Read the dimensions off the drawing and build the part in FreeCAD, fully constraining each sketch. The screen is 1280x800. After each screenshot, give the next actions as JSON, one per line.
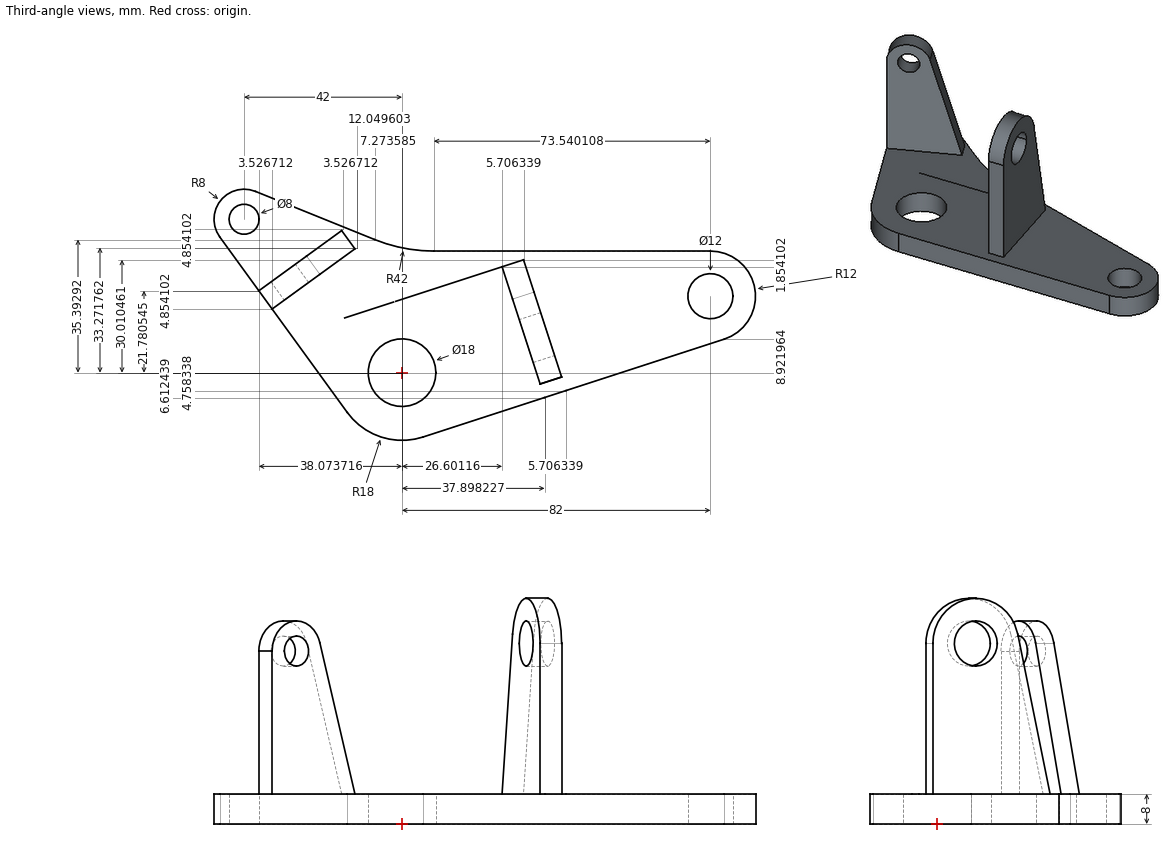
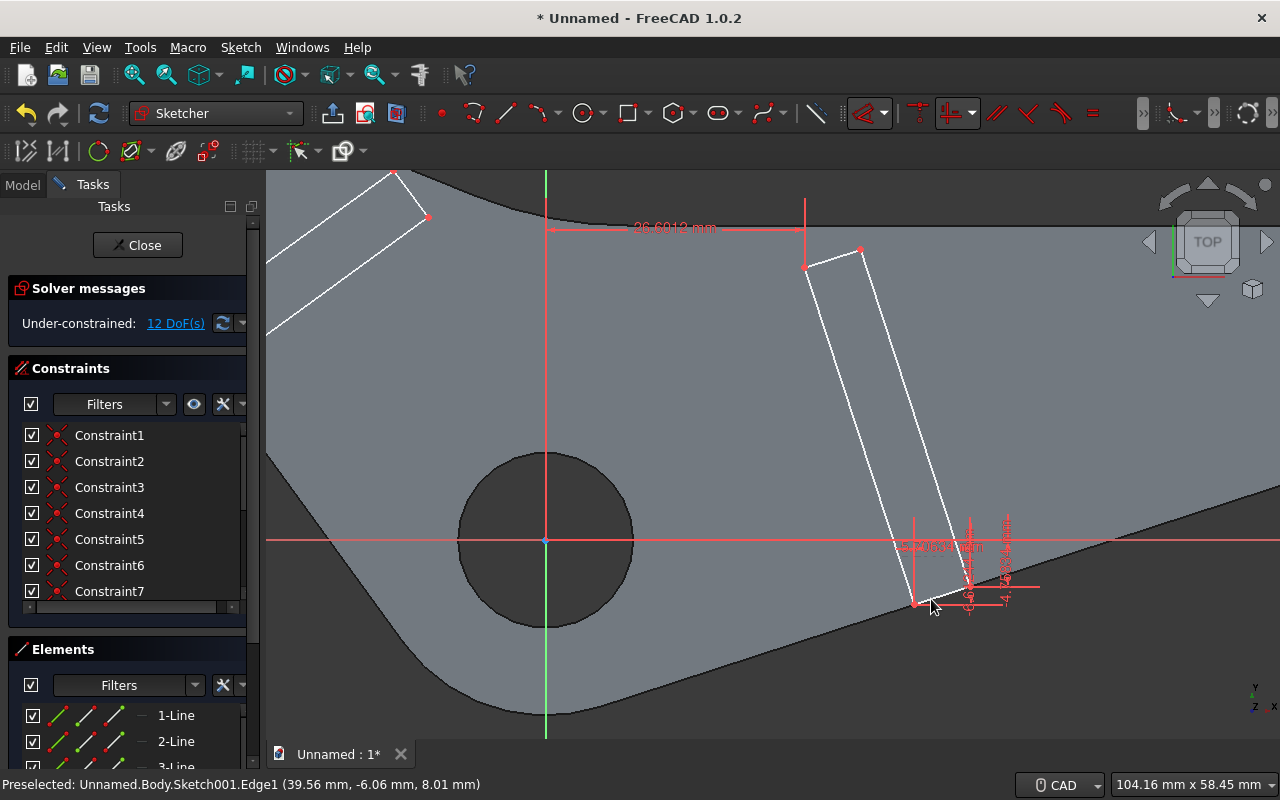
{"action": "left_click", "coordinate": [844, 255]}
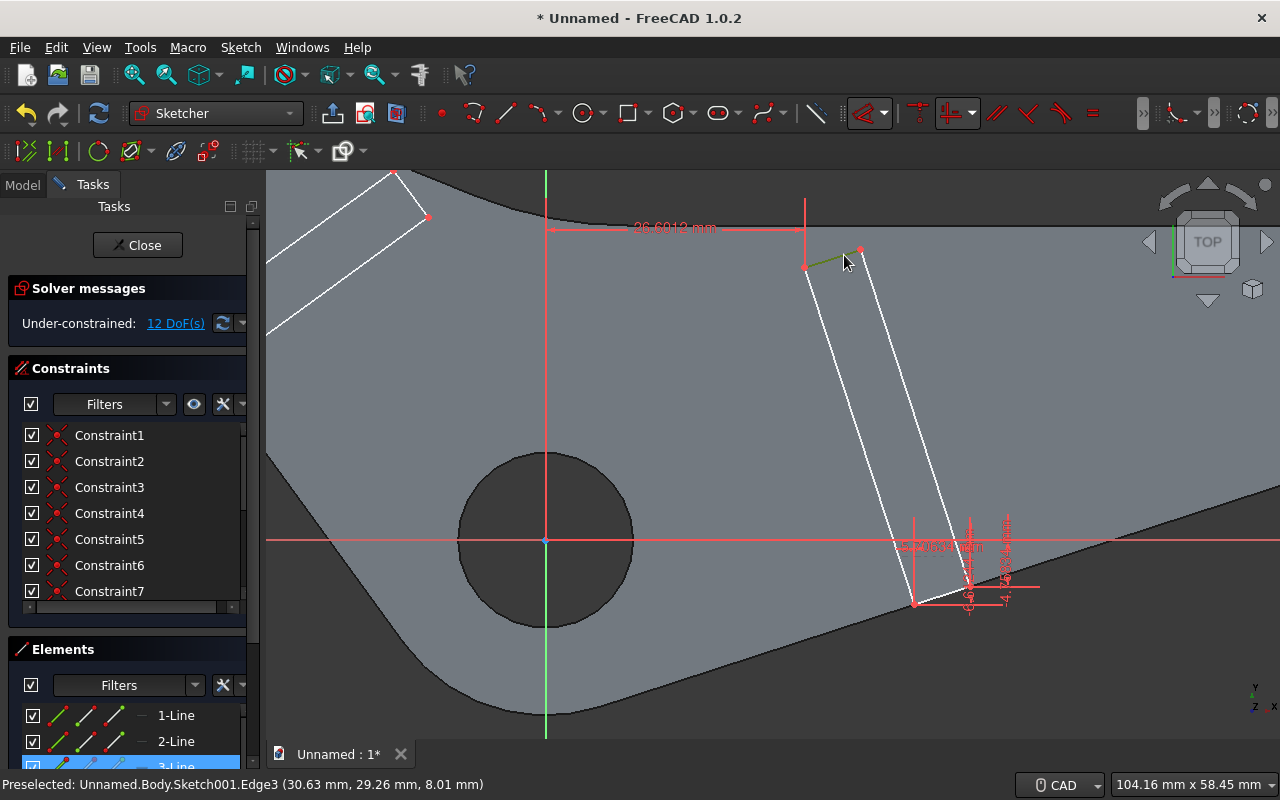
{"action": "key", "text": "l"}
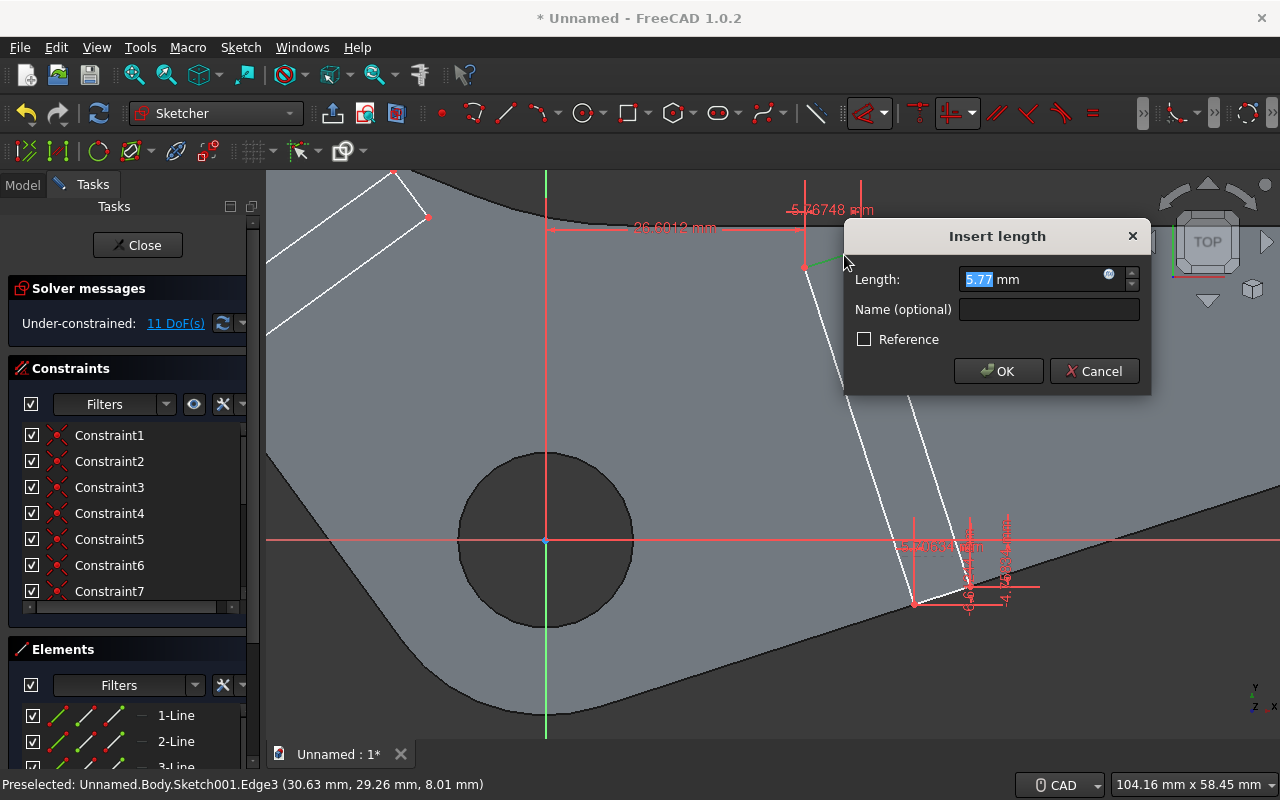
{"action": "type", "text": "5.706339"}
{"action": "key", "text": "Return"}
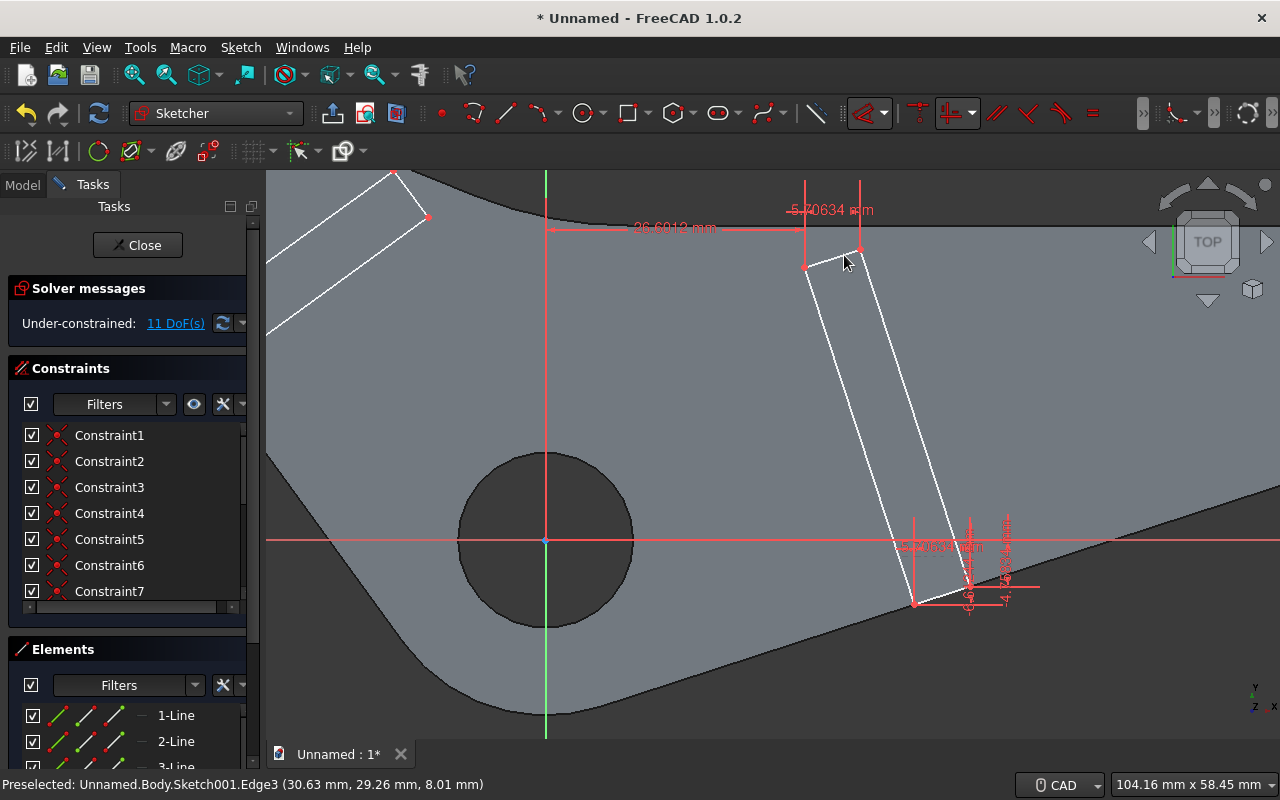
{"action": "scroll", "coordinate": [843, 255], "scroll_direction": "up", "scroll_amount": 4}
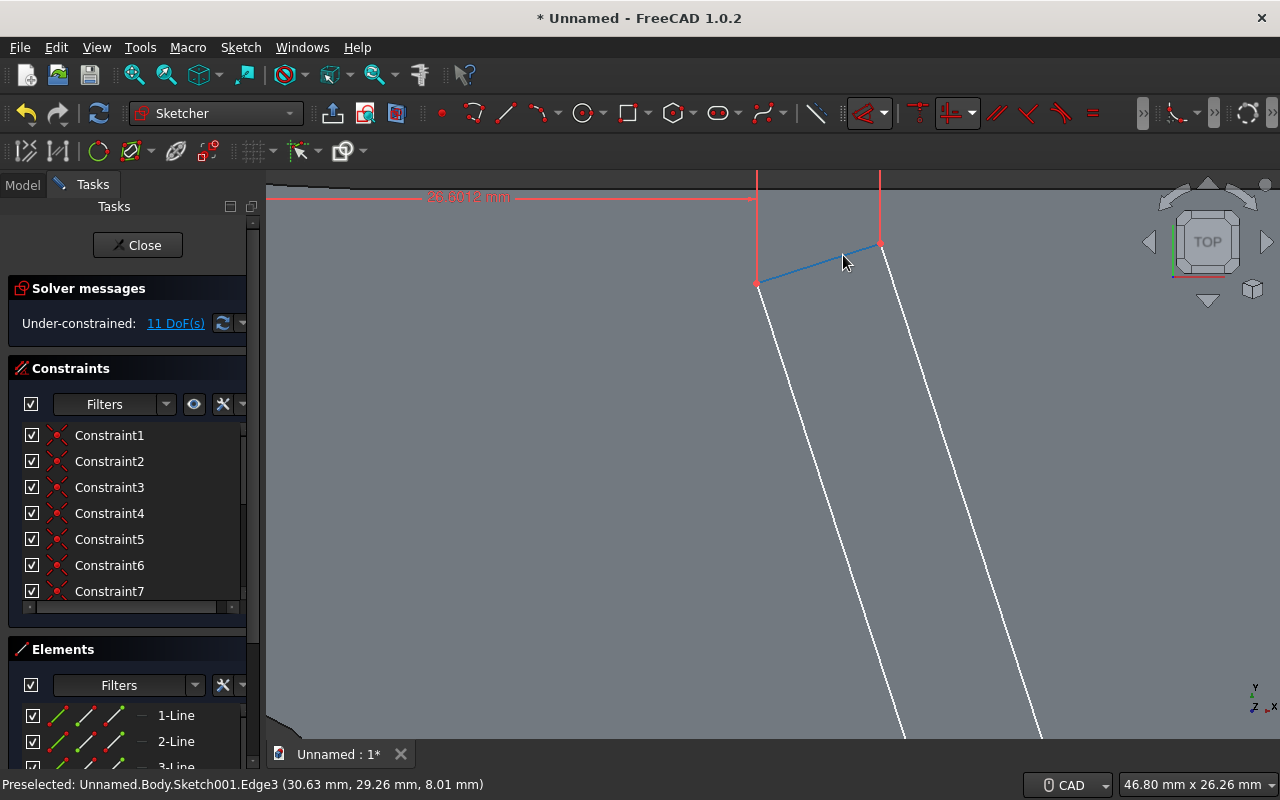
{"action": "left_click", "coordinate": [843, 256]}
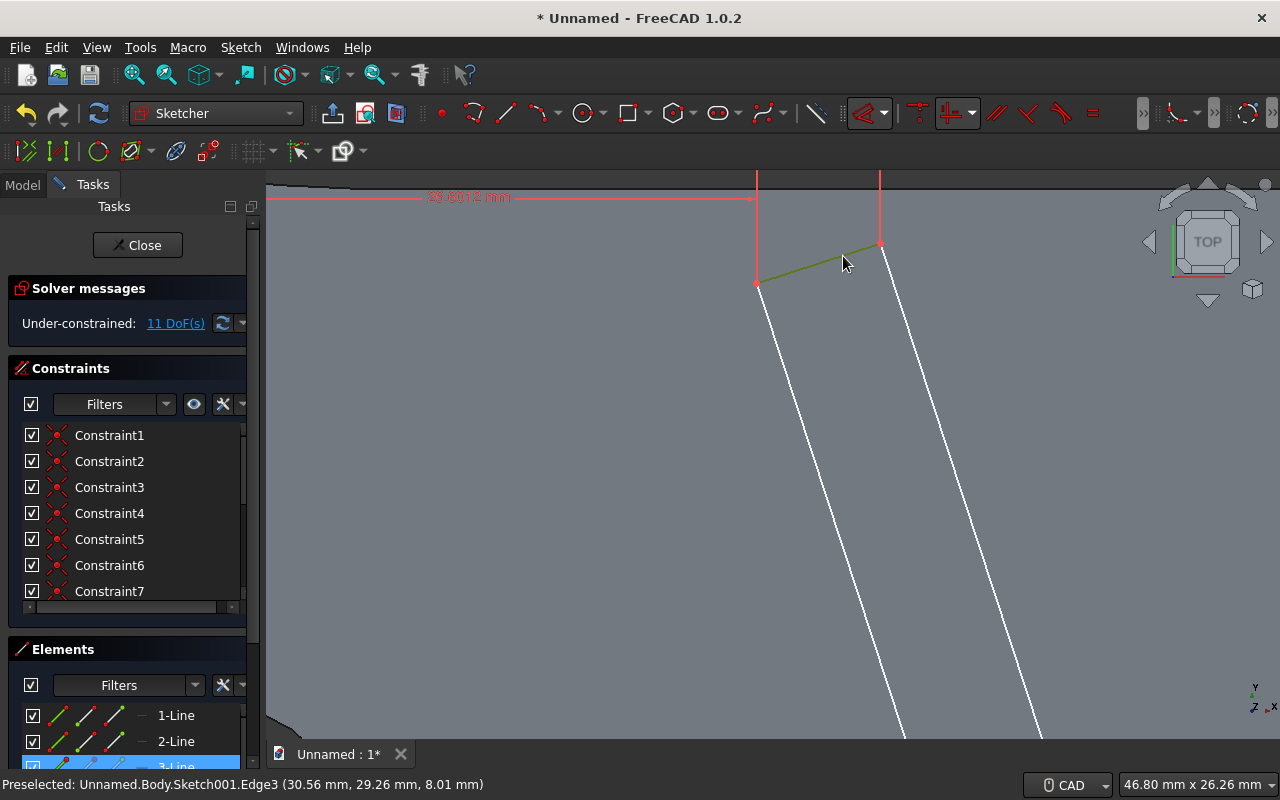
{"action": "key", "text": "i"}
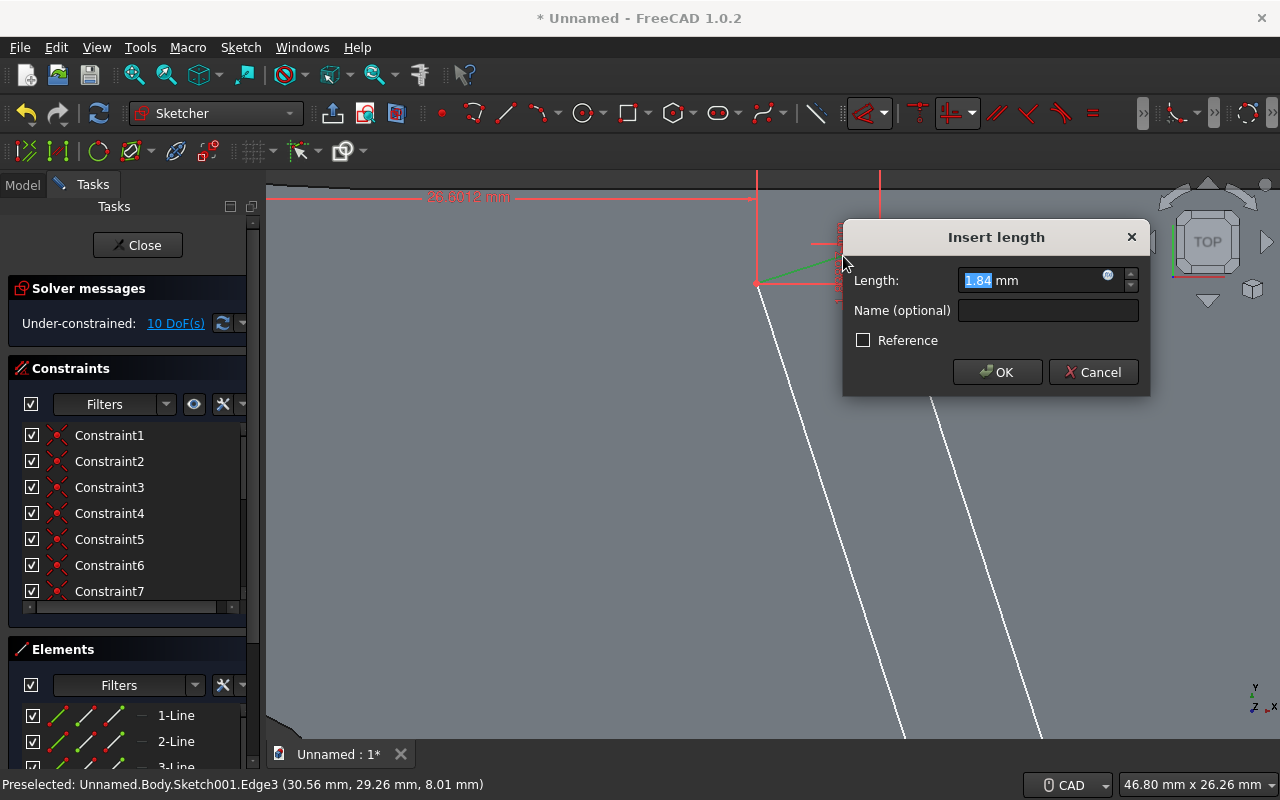
{"action": "type", "text": "1.854102"}
{"action": "key", "text": "Return"}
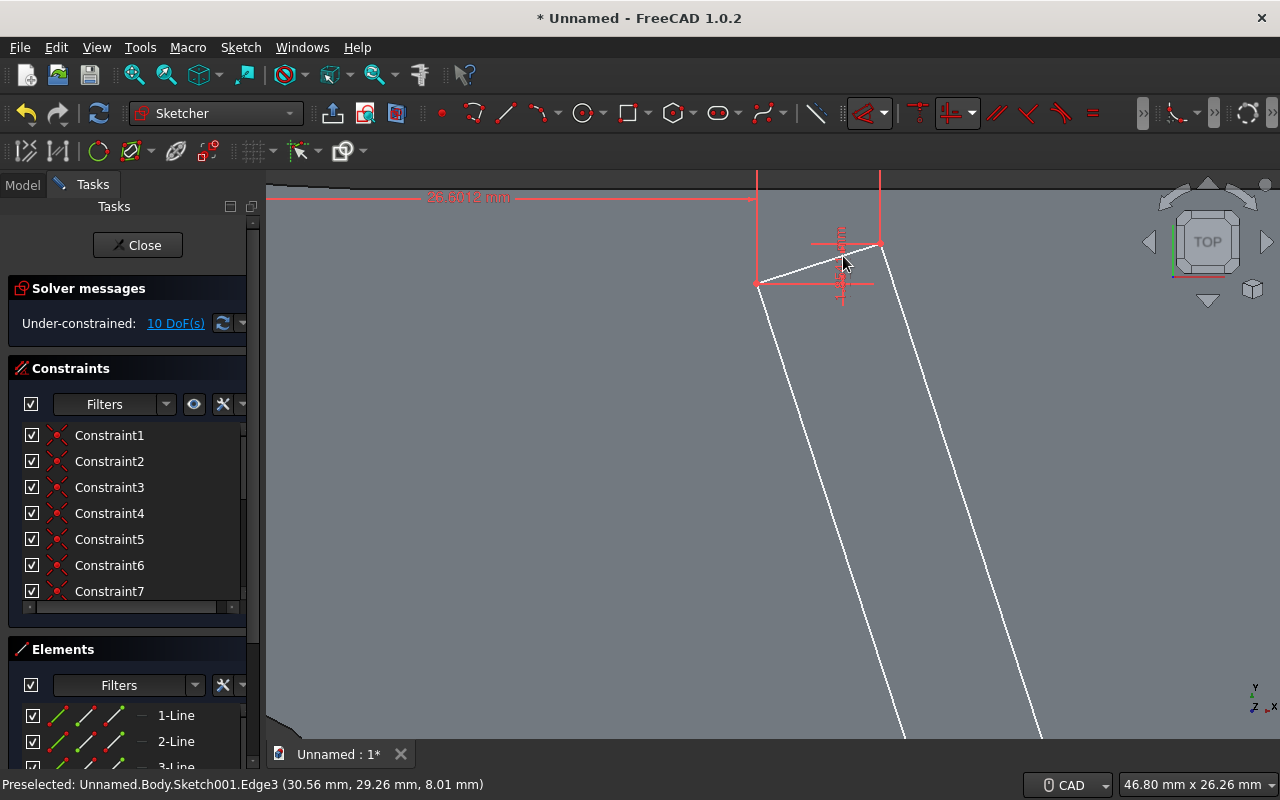
{"action": "scroll", "coordinate": [905, 414], "scroll_direction": "down", "scroll_amount": 6}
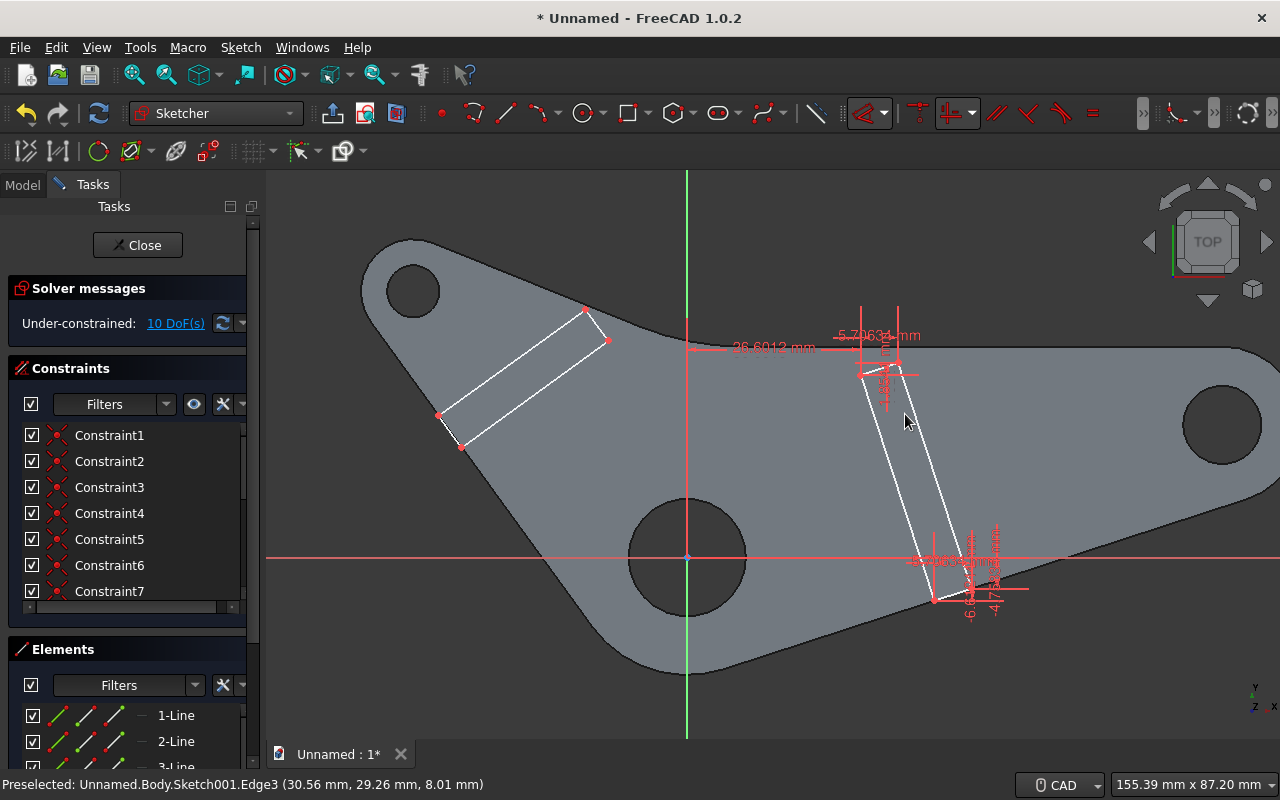
{"action": "scroll", "coordinate": [602, 332], "scroll_direction": "up", "scroll_amount": 3}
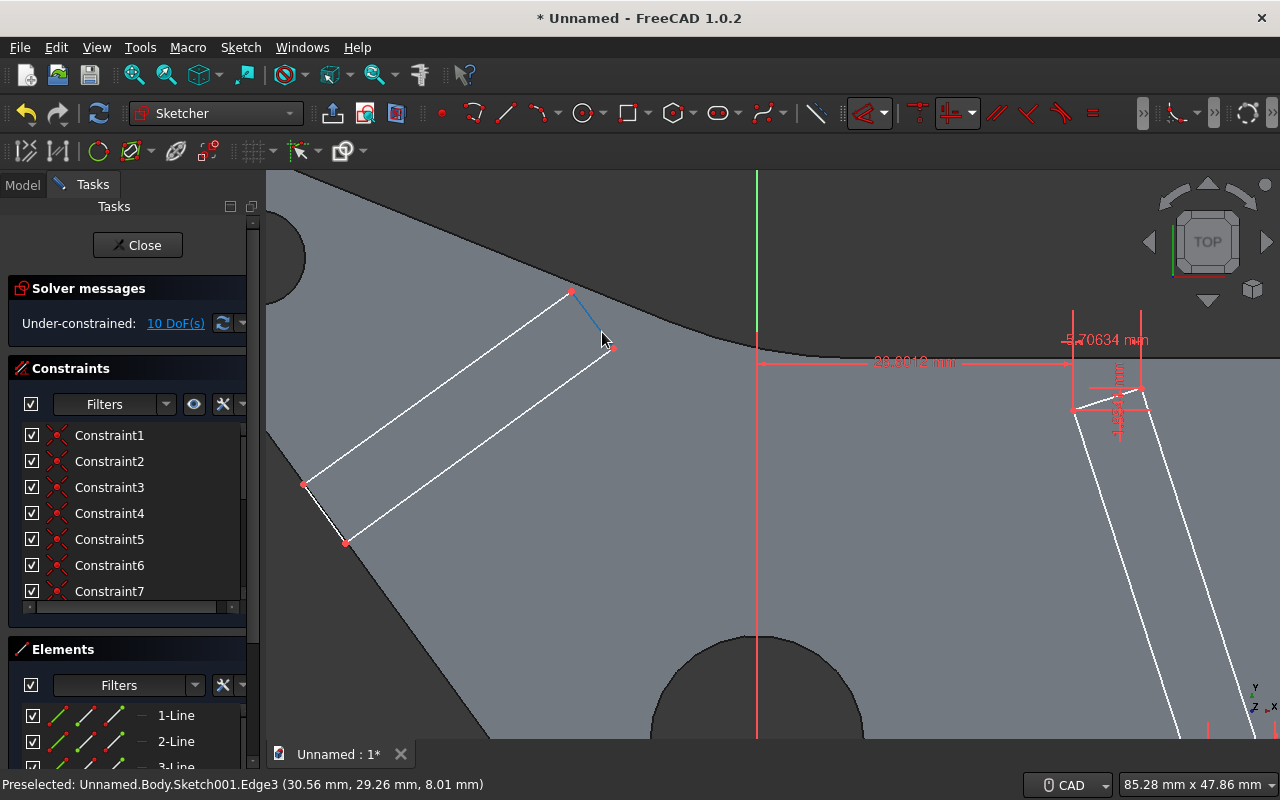
{"action": "left_click", "coordinate": [601, 331]}